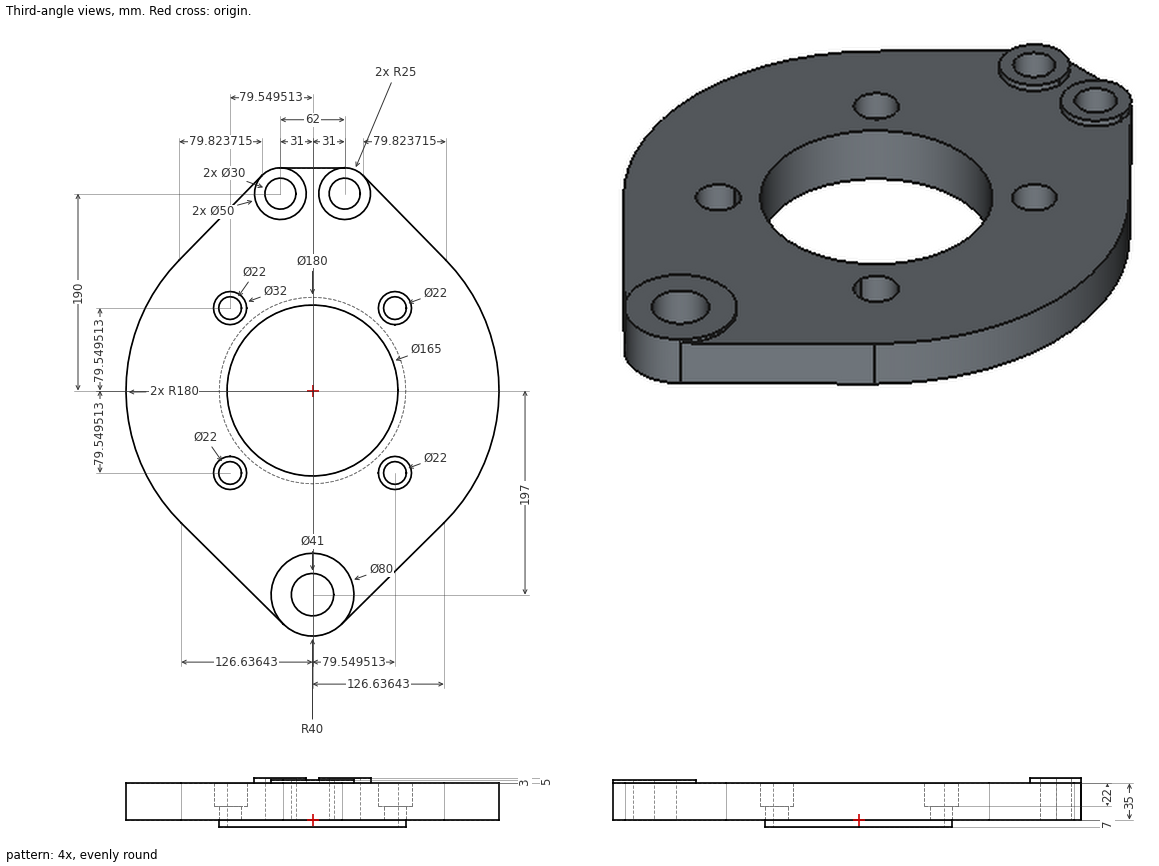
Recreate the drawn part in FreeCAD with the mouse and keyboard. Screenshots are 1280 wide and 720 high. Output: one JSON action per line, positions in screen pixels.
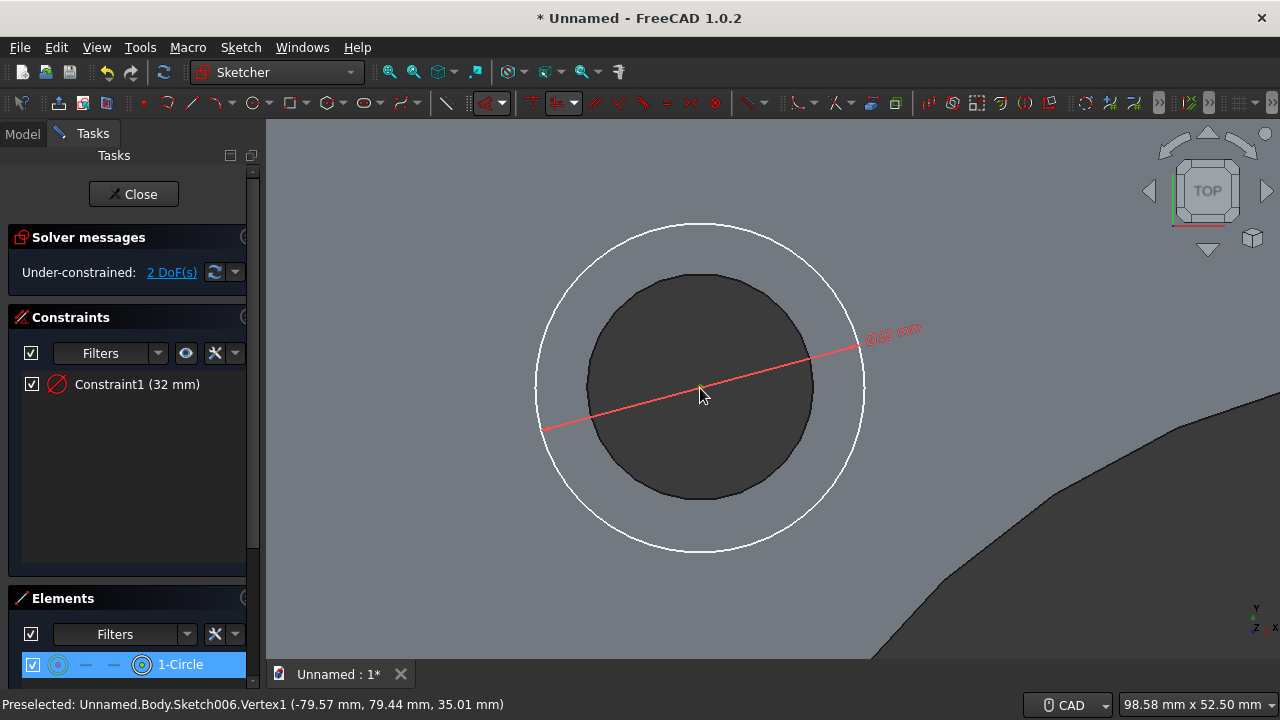
{"action": "key", "text": "l"}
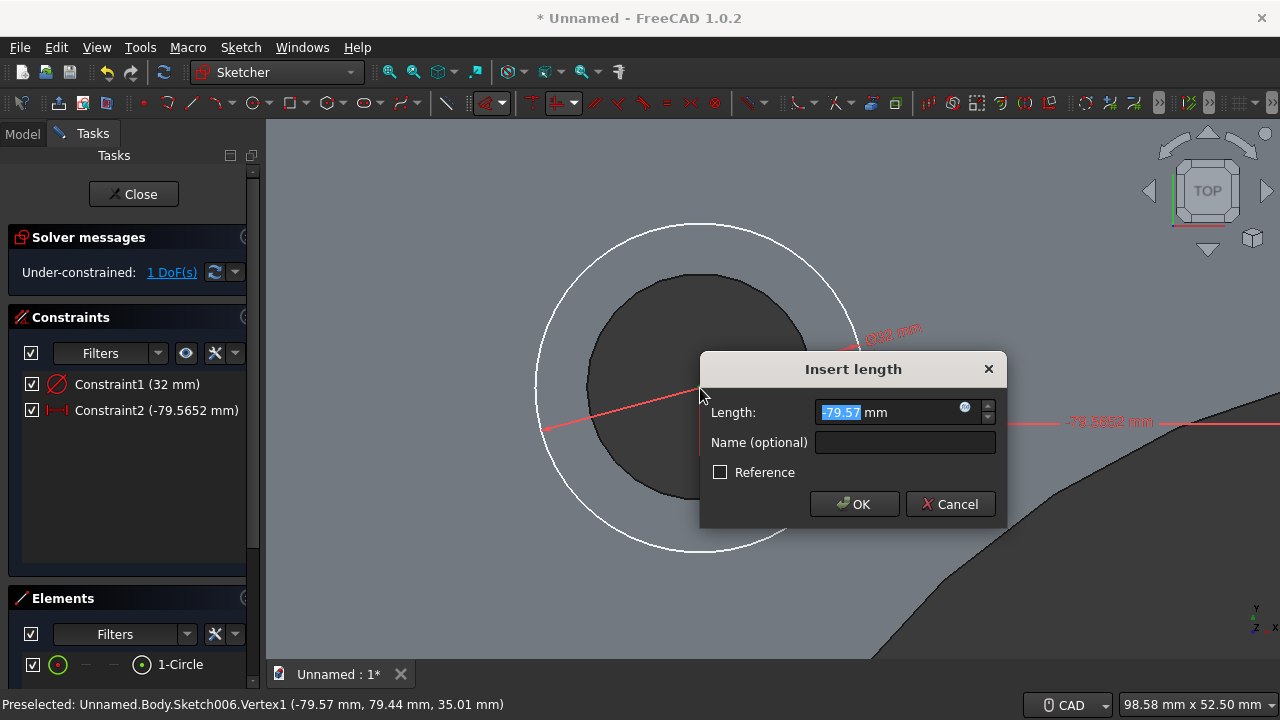
{"action": "type", "text": "-79.549513"}
{"action": "key", "text": "Return"}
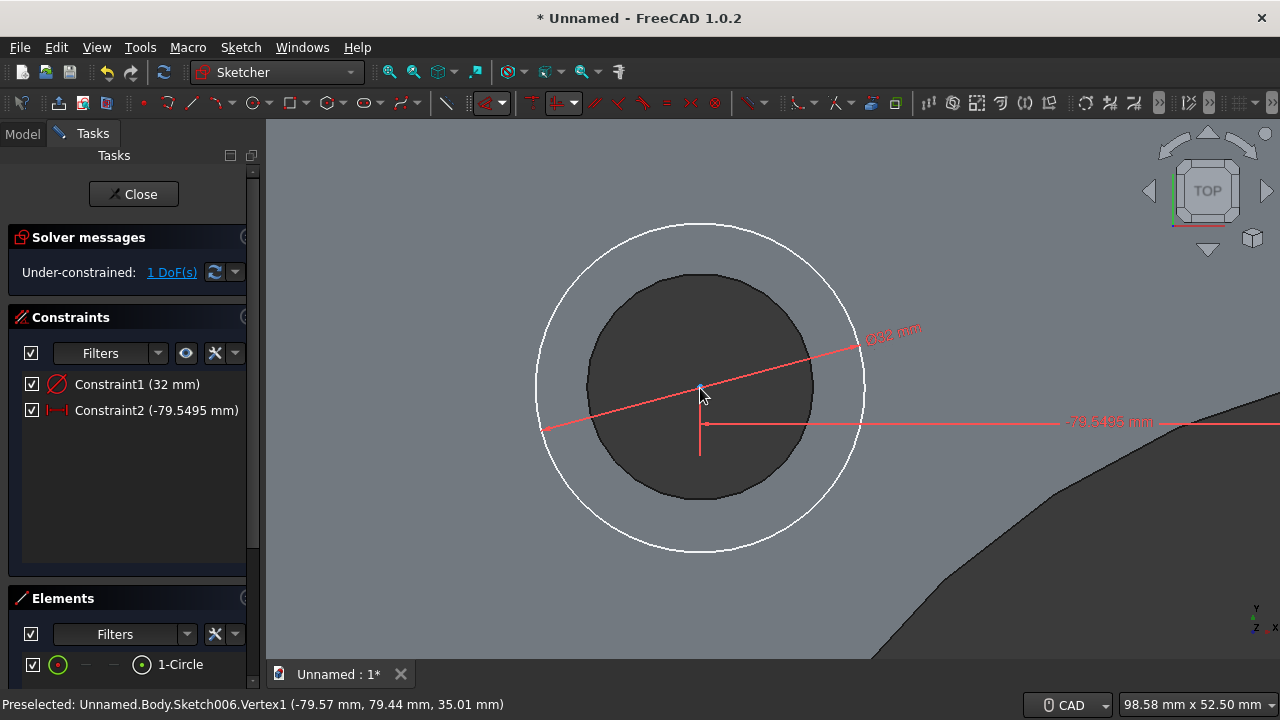
{"action": "left_click", "coordinate": [700, 388]}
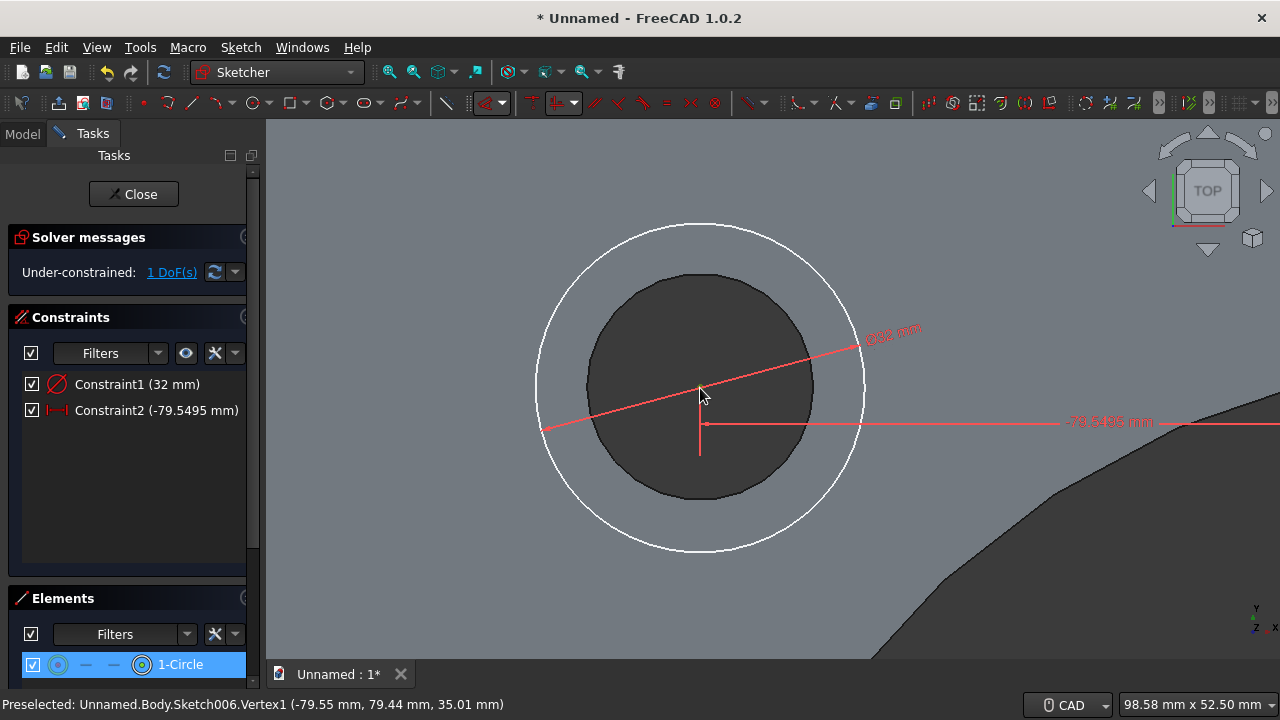
{"action": "key", "text": "i"}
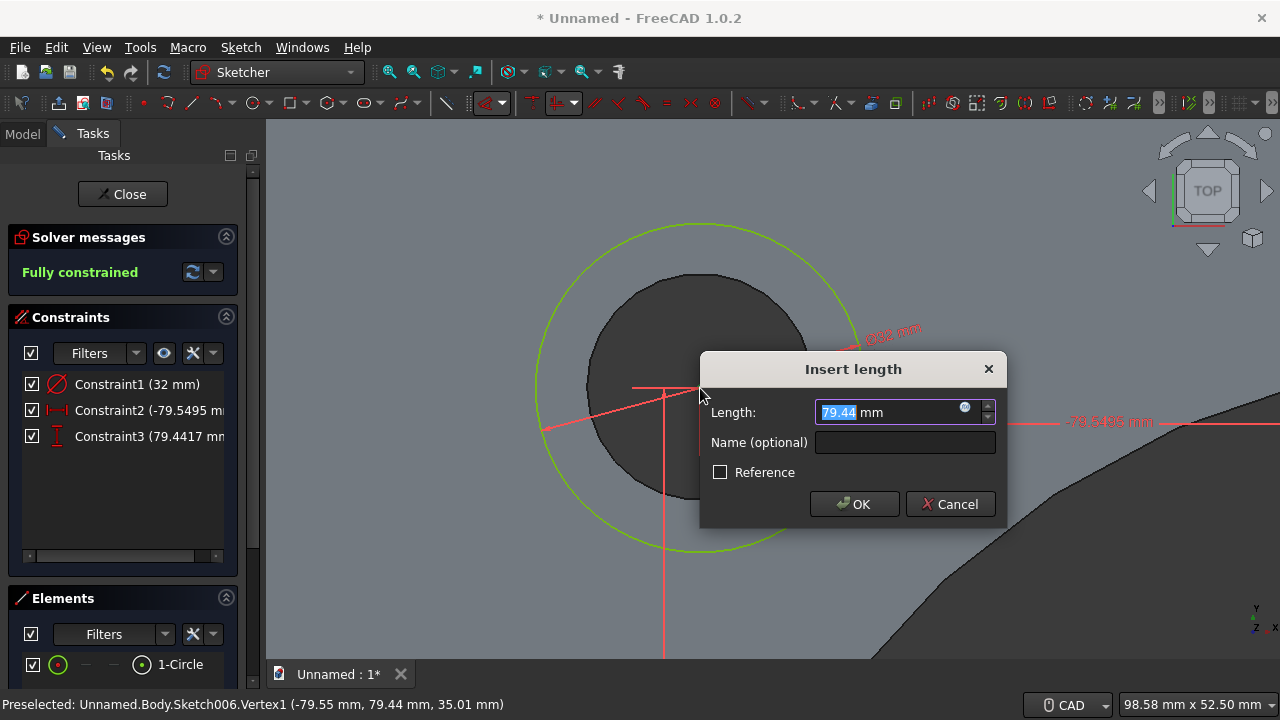
{"action": "type", "text": "79.549513"}
{"action": "key", "text": "Return"}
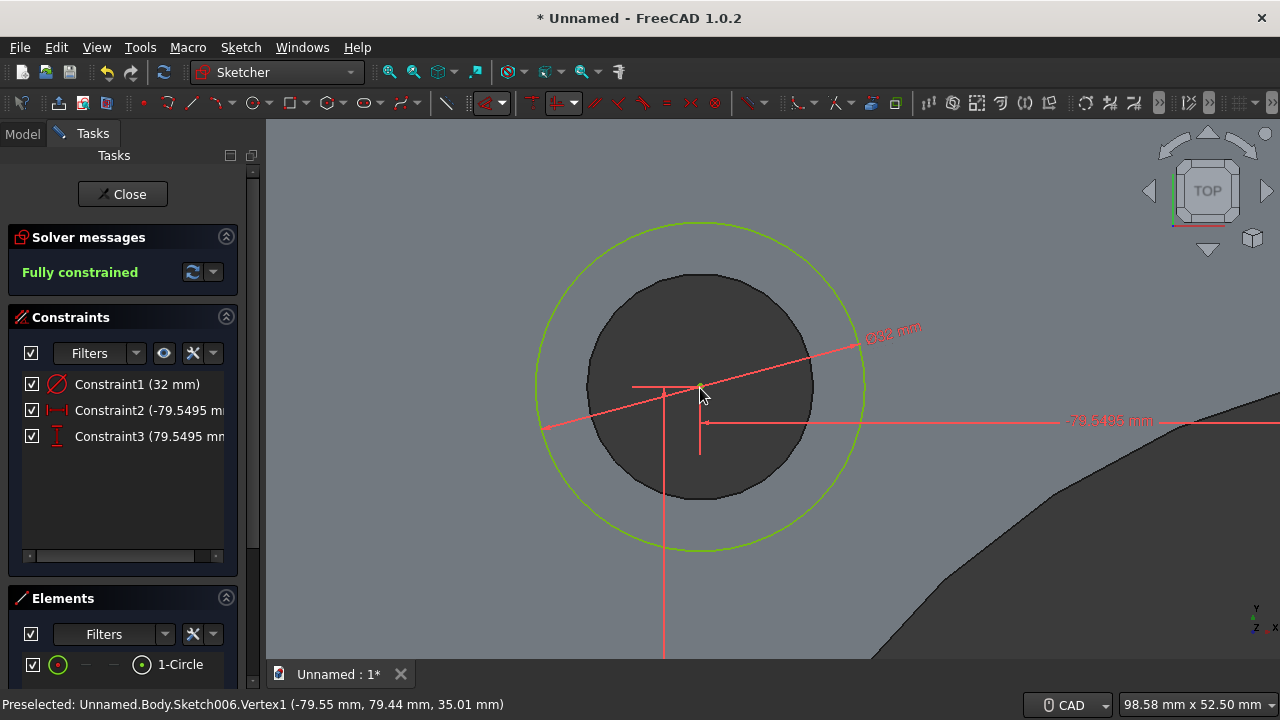
{"action": "left_click", "coordinate": [123, 194]}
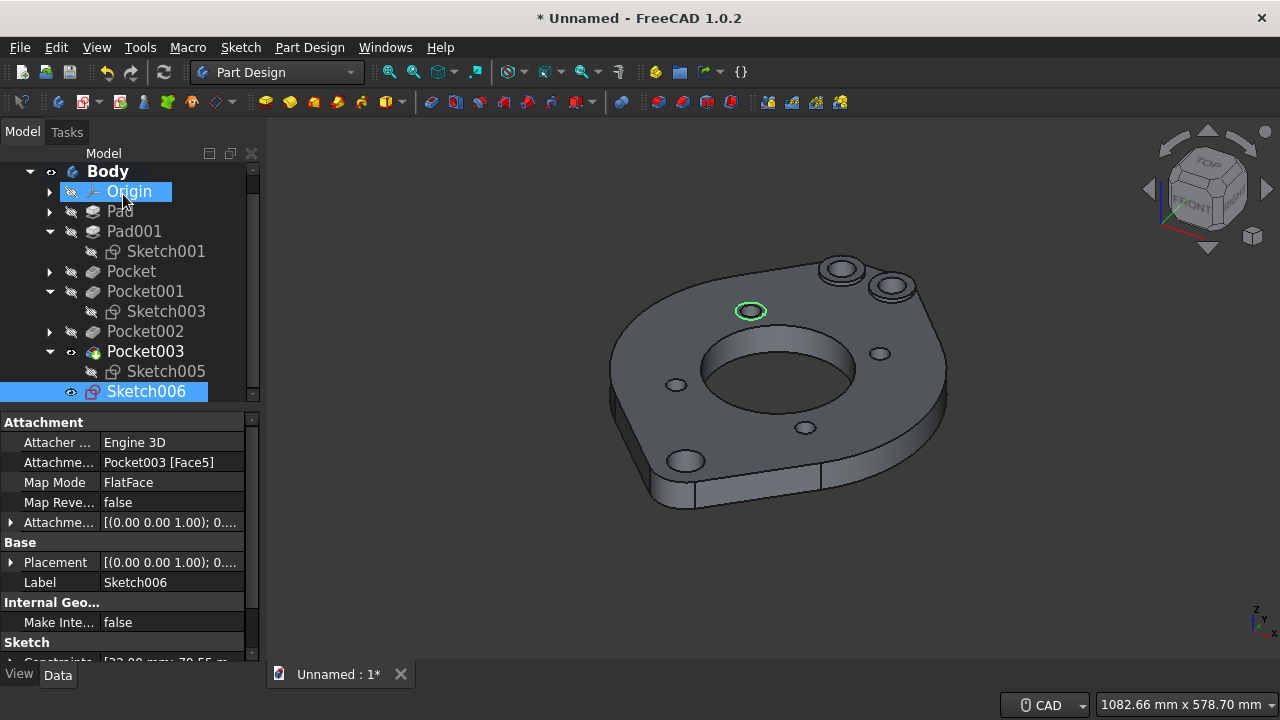
{"action": "left_click", "coordinate": [432, 102]}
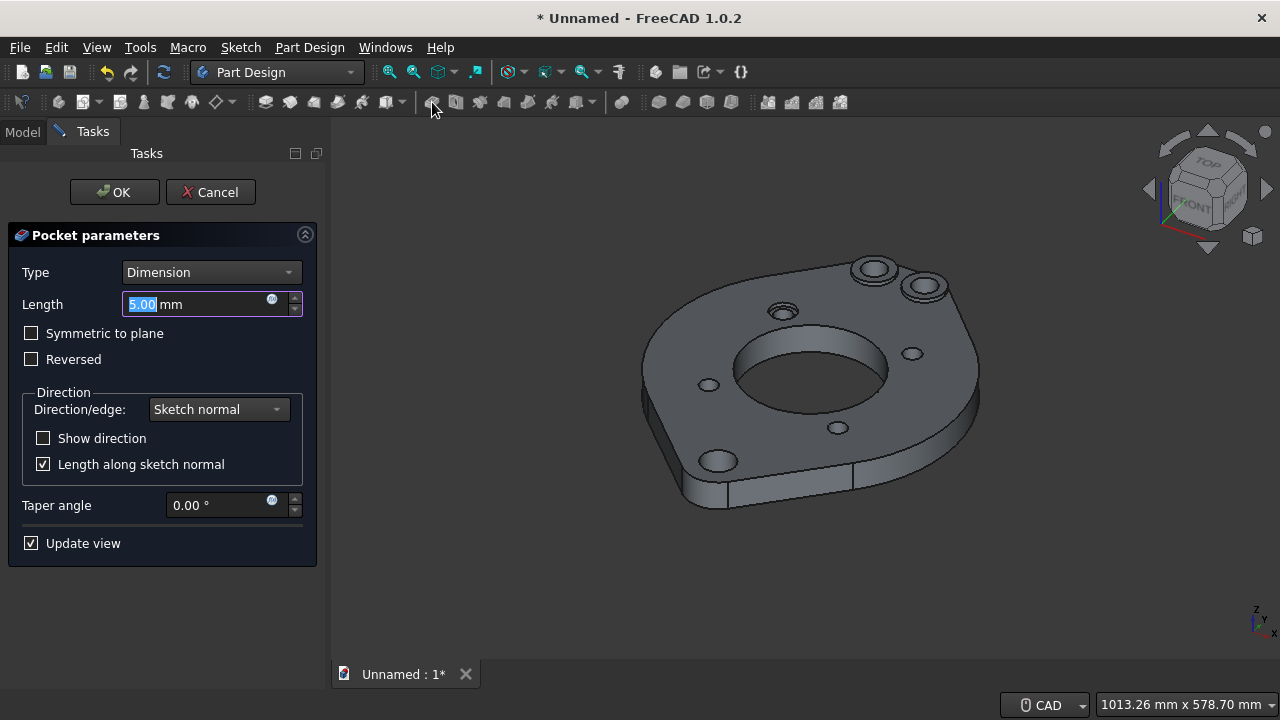
{"action": "type", "text": "22"}
{"action": "key", "text": "Tab"}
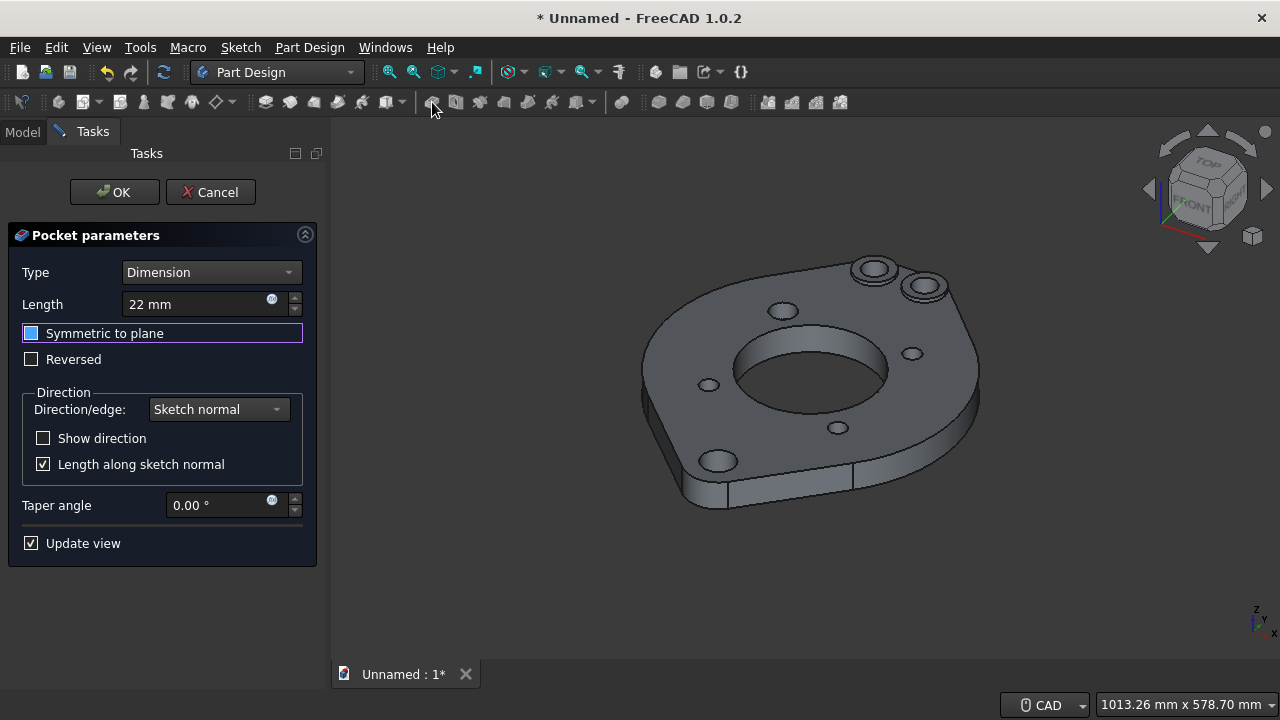
{"action": "left_click", "coordinate": [115, 192]}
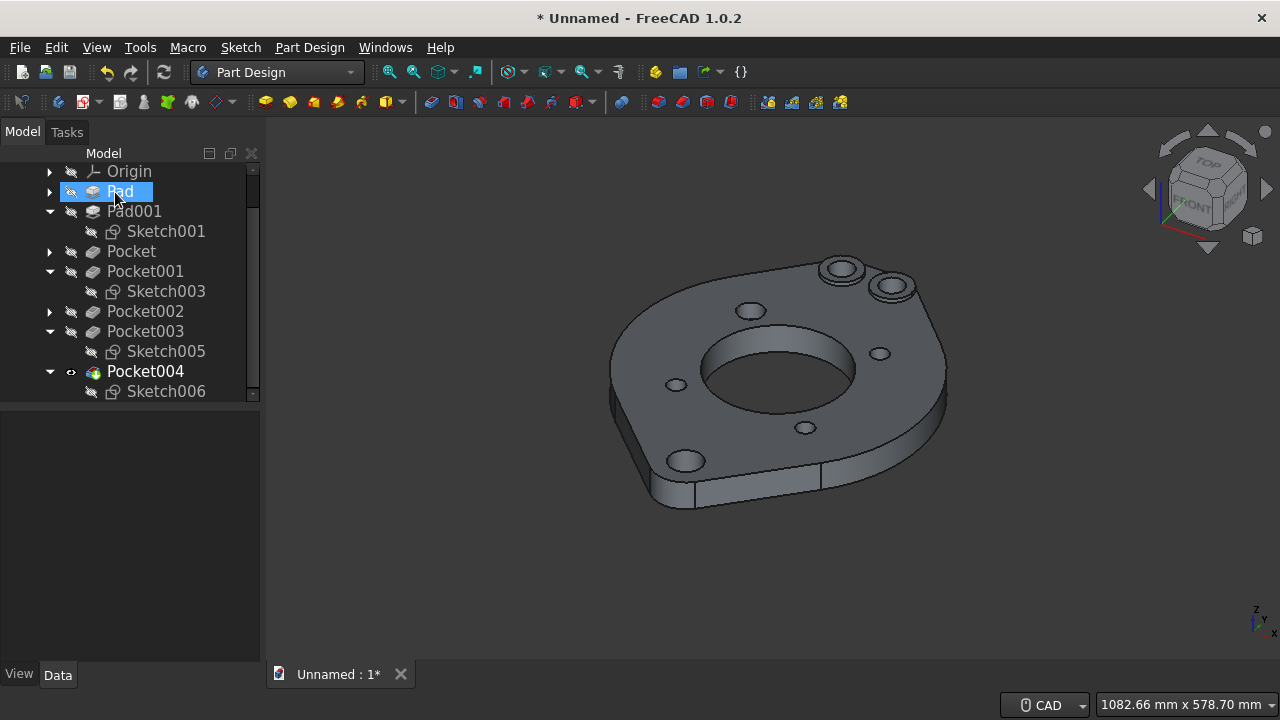
{"action": "left_click", "coordinate": [116, 372]}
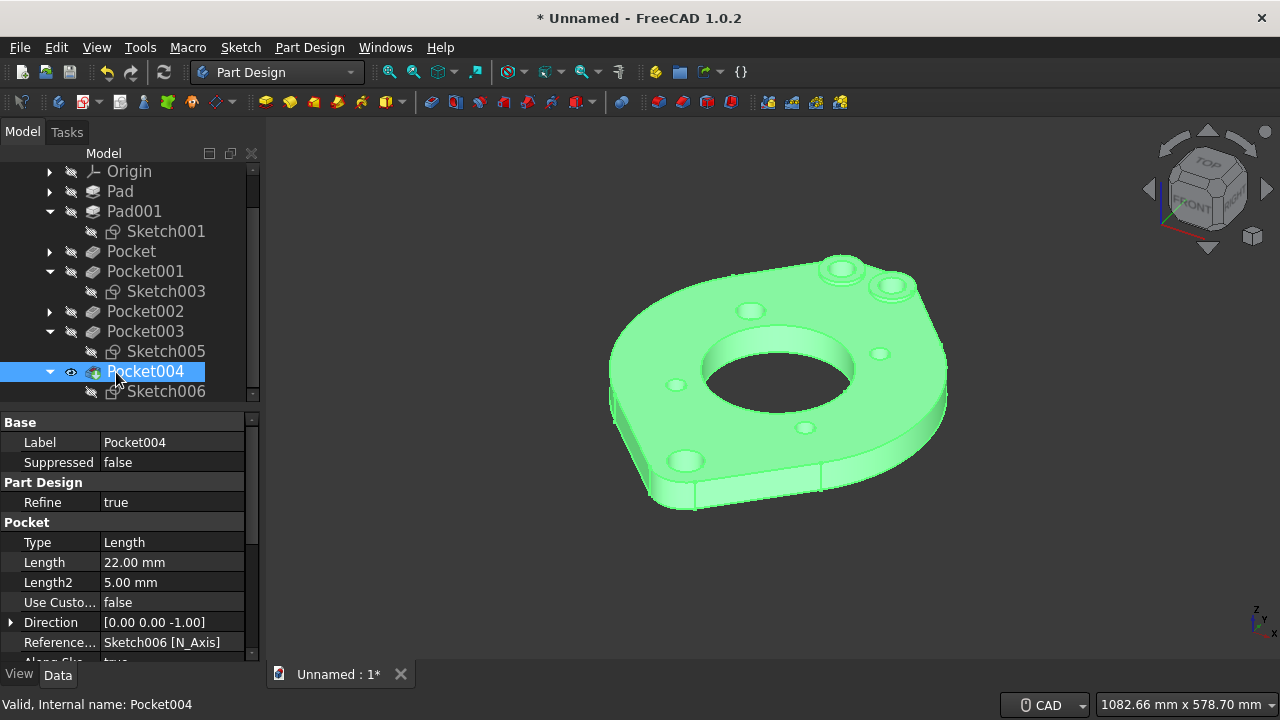
{"action": "left_click", "coordinate": [816, 102]}